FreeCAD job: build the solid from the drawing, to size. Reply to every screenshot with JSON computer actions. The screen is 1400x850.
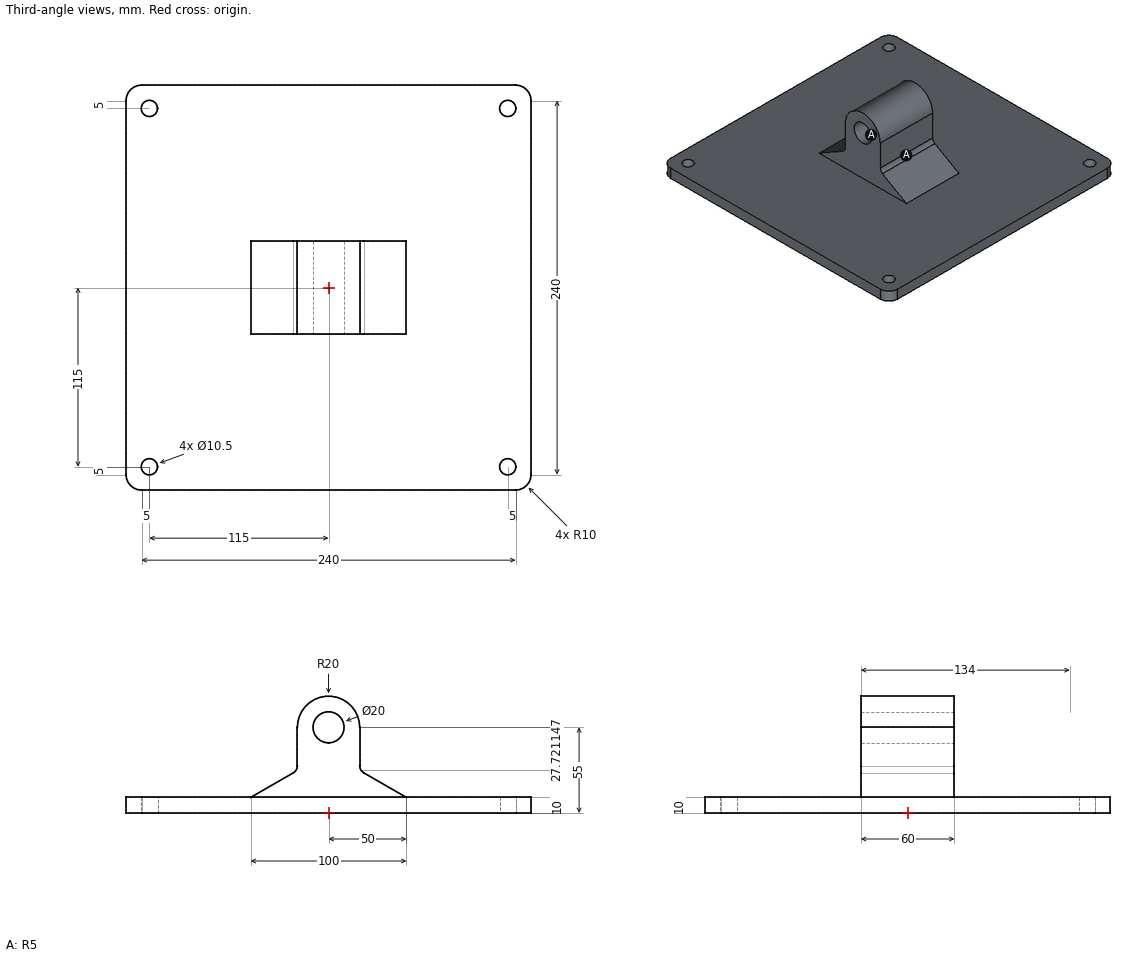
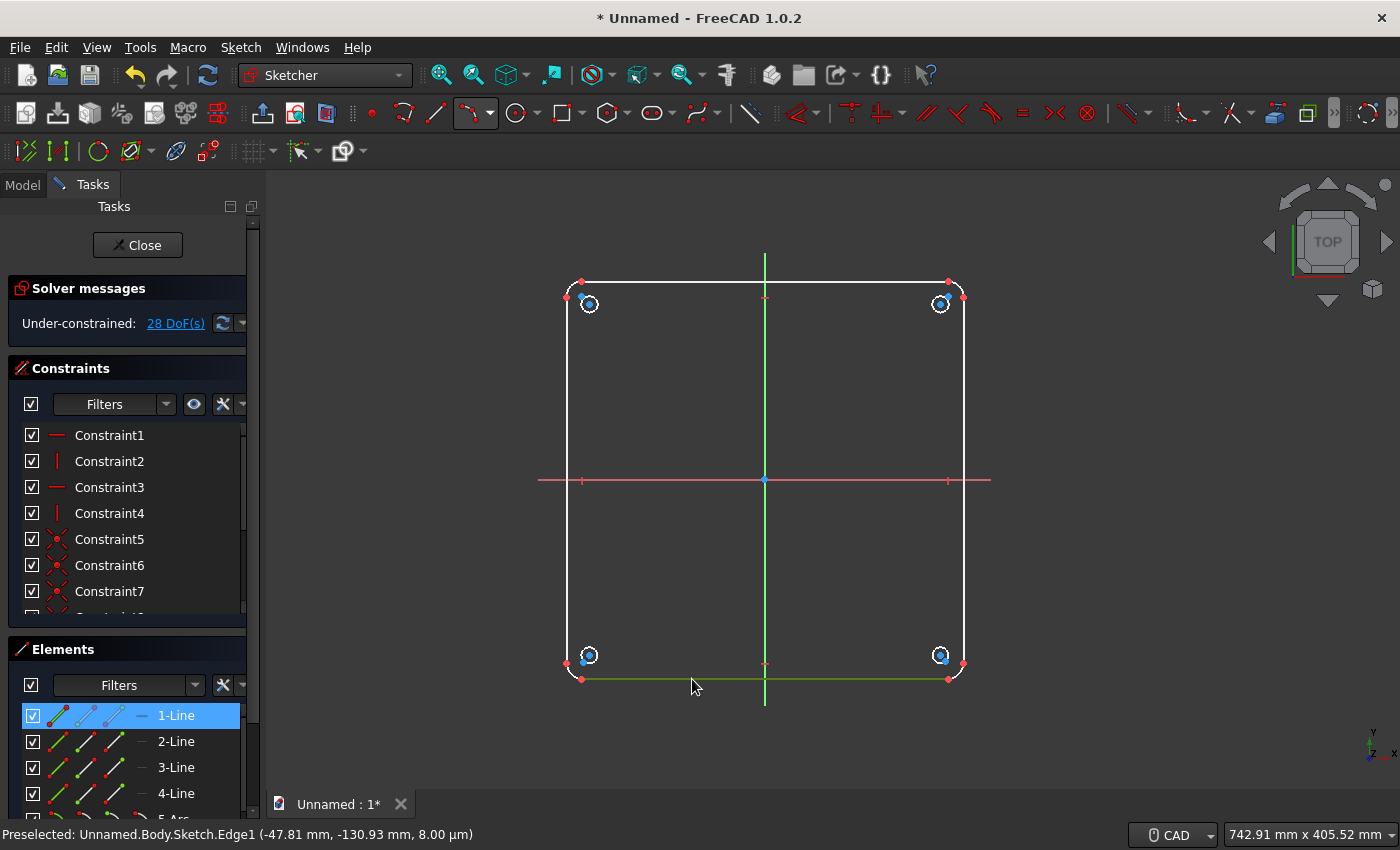
{"action": "left_click", "coordinate": [959, 674]}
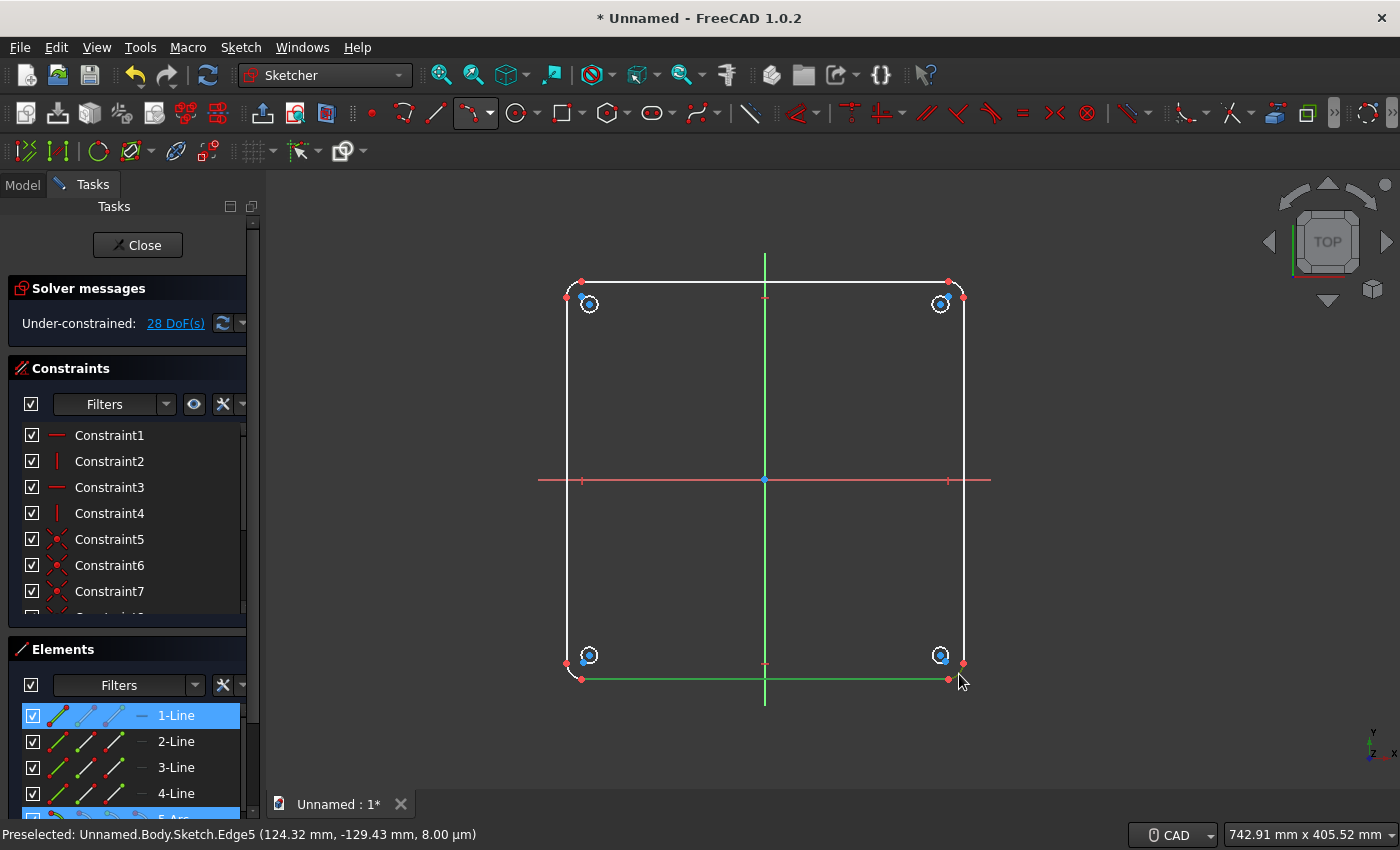
{"action": "left_click", "coordinate": [992, 114]}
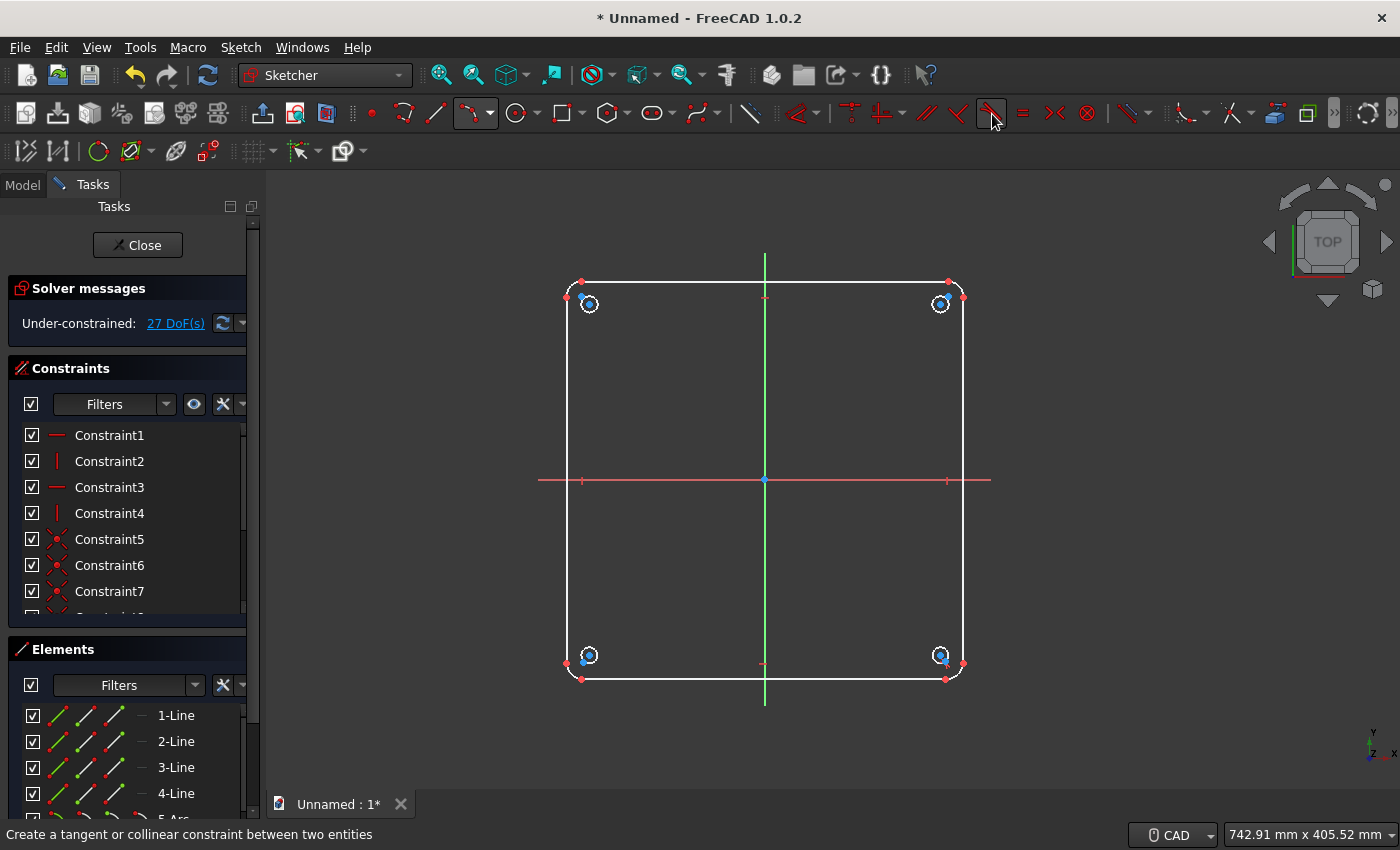
{"action": "left_click", "coordinate": [691, 679]}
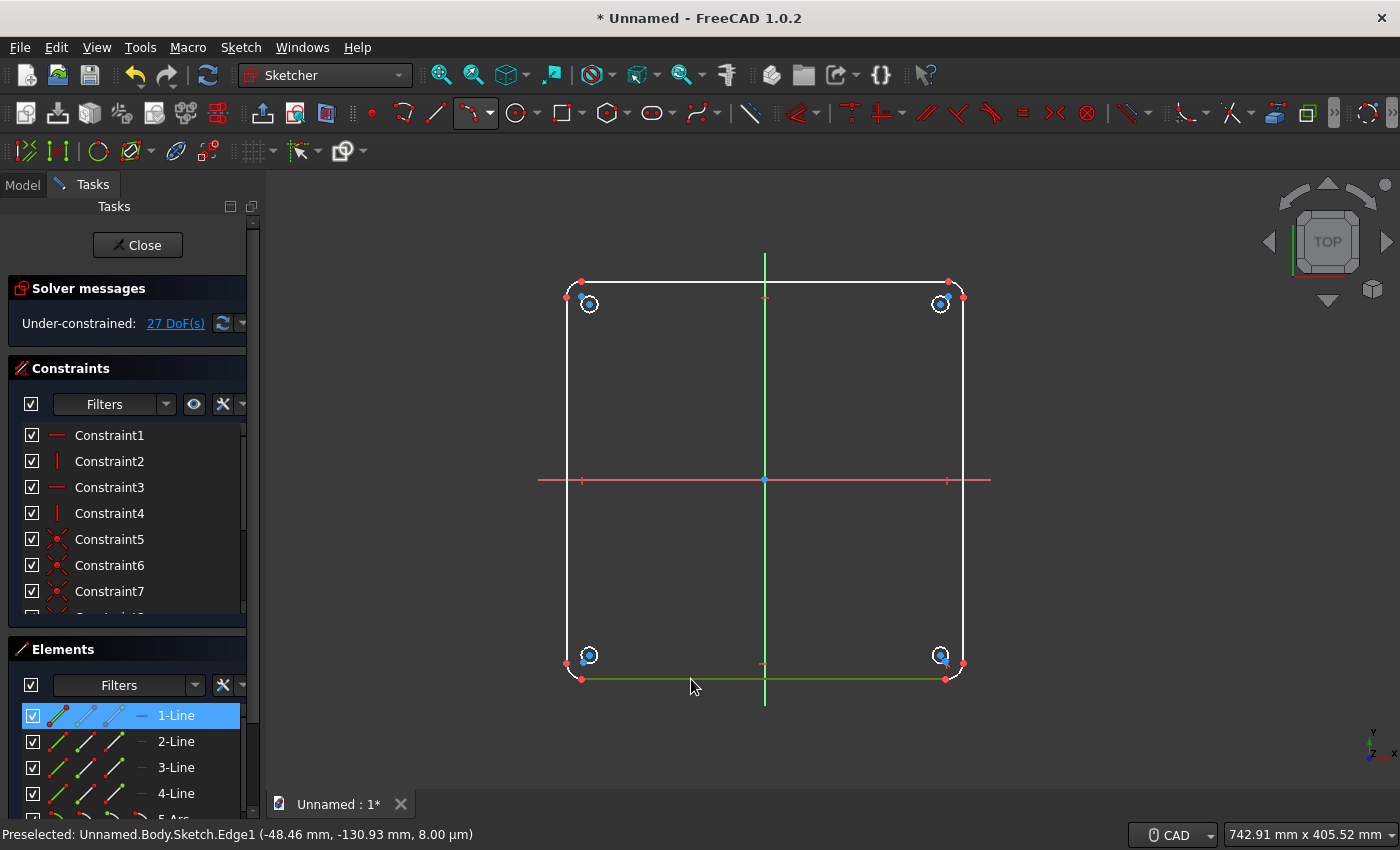
{"action": "left_click", "coordinate": [571, 674]}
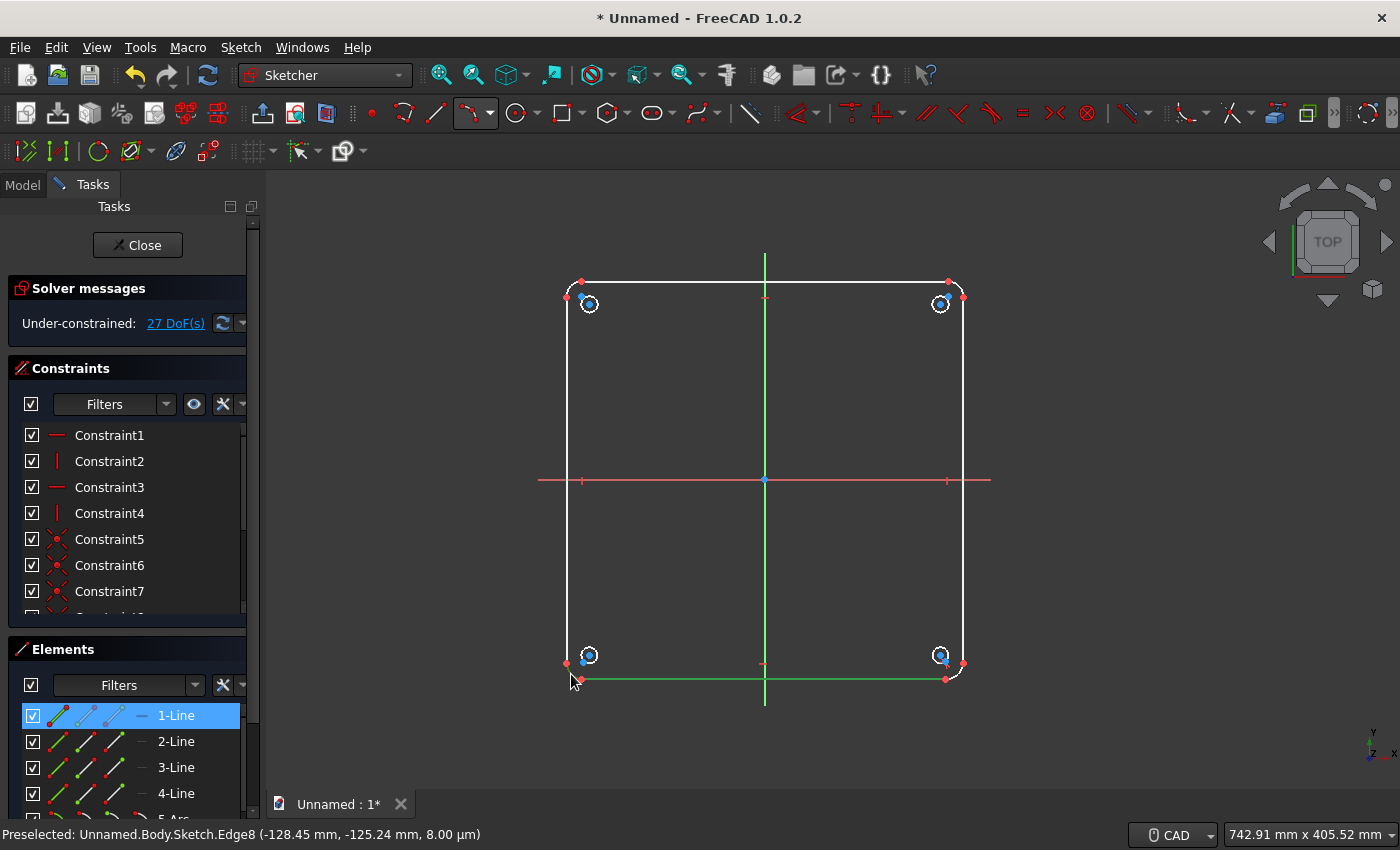
{"action": "left_click", "coordinate": [992, 114]}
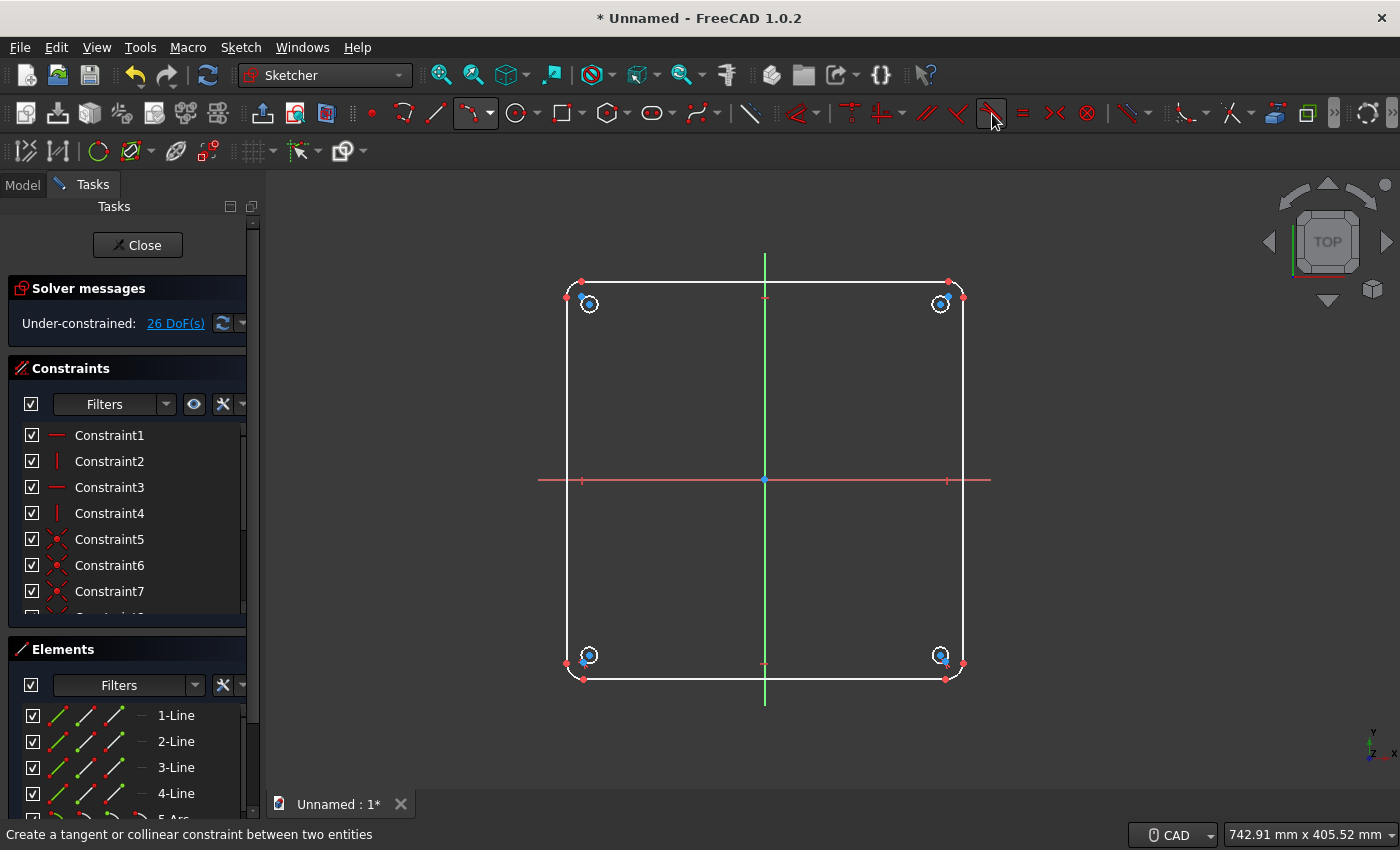
{"action": "left_click", "coordinate": [963, 554]}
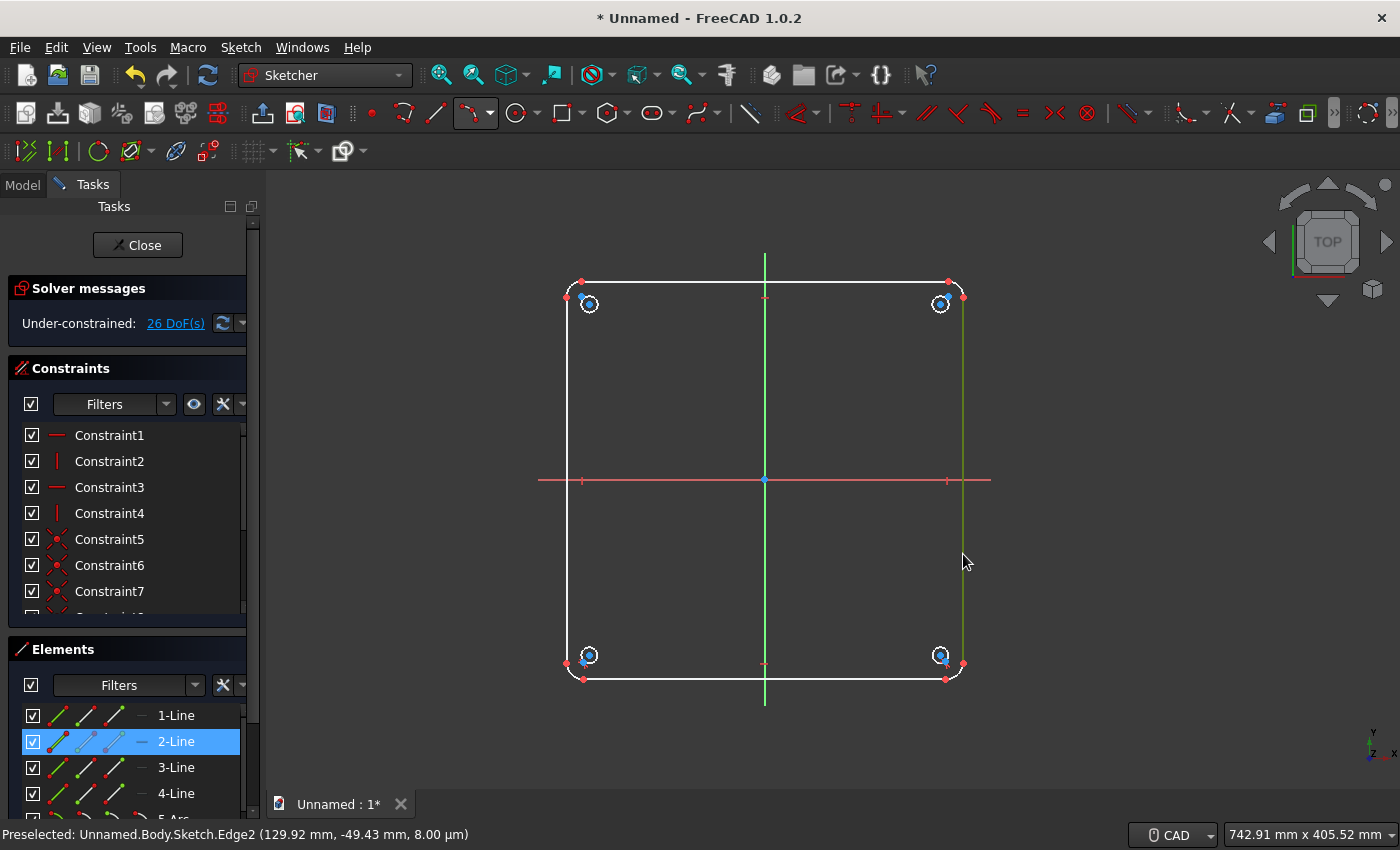
{"action": "left_click", "coordinate": [957, 675]}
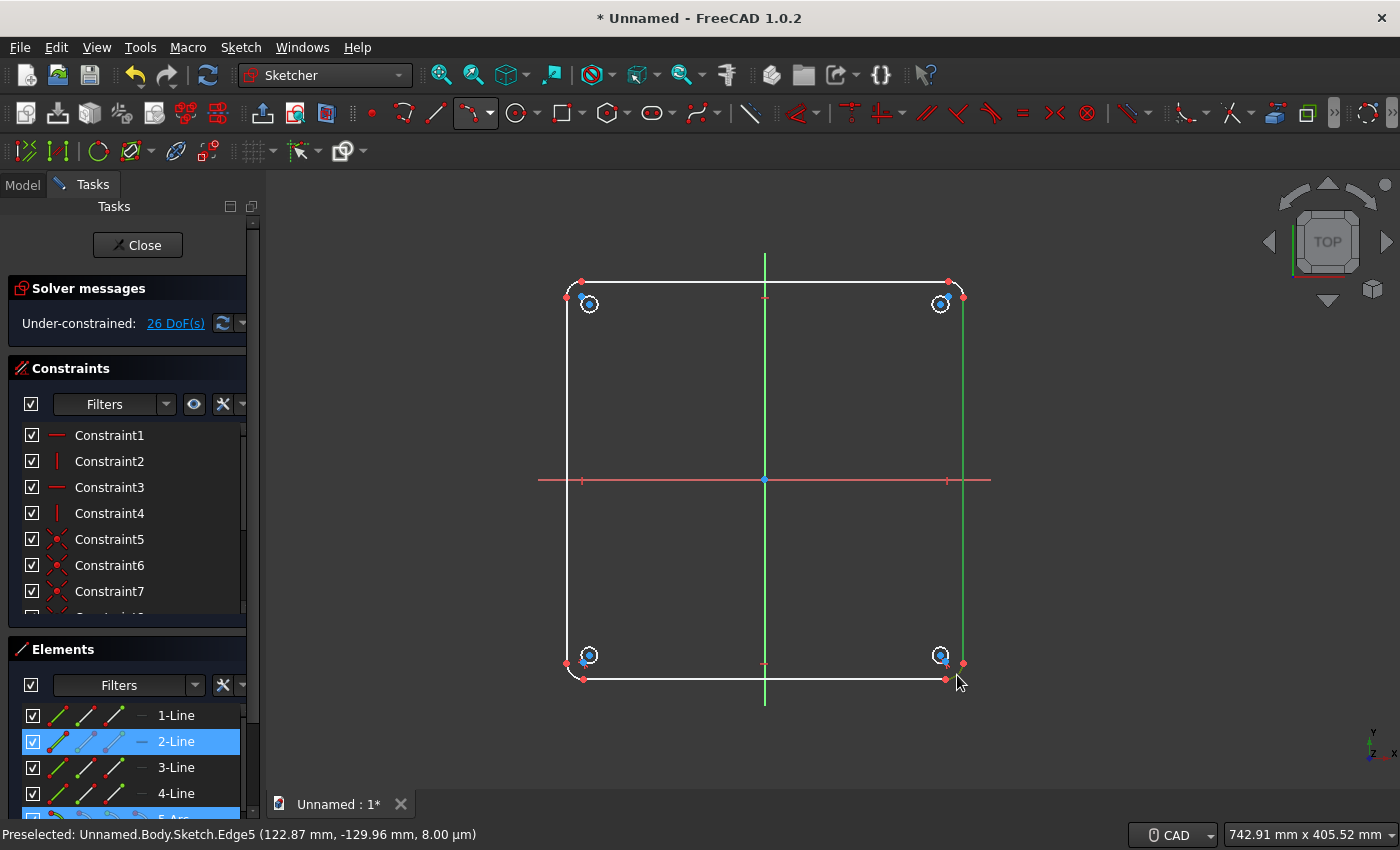
{"action": "left_click", "coordinate": [992, 114]}